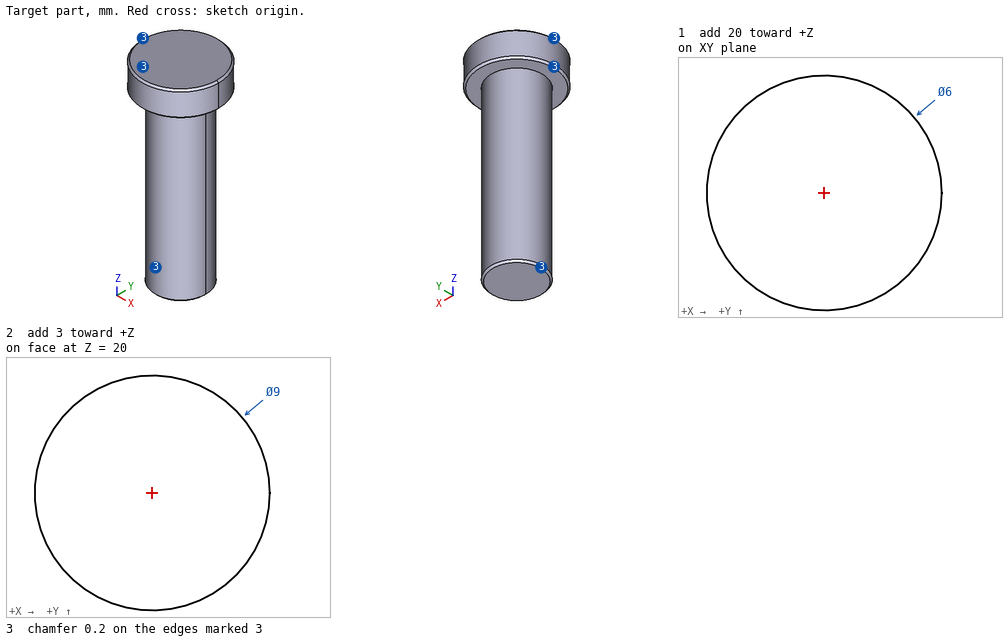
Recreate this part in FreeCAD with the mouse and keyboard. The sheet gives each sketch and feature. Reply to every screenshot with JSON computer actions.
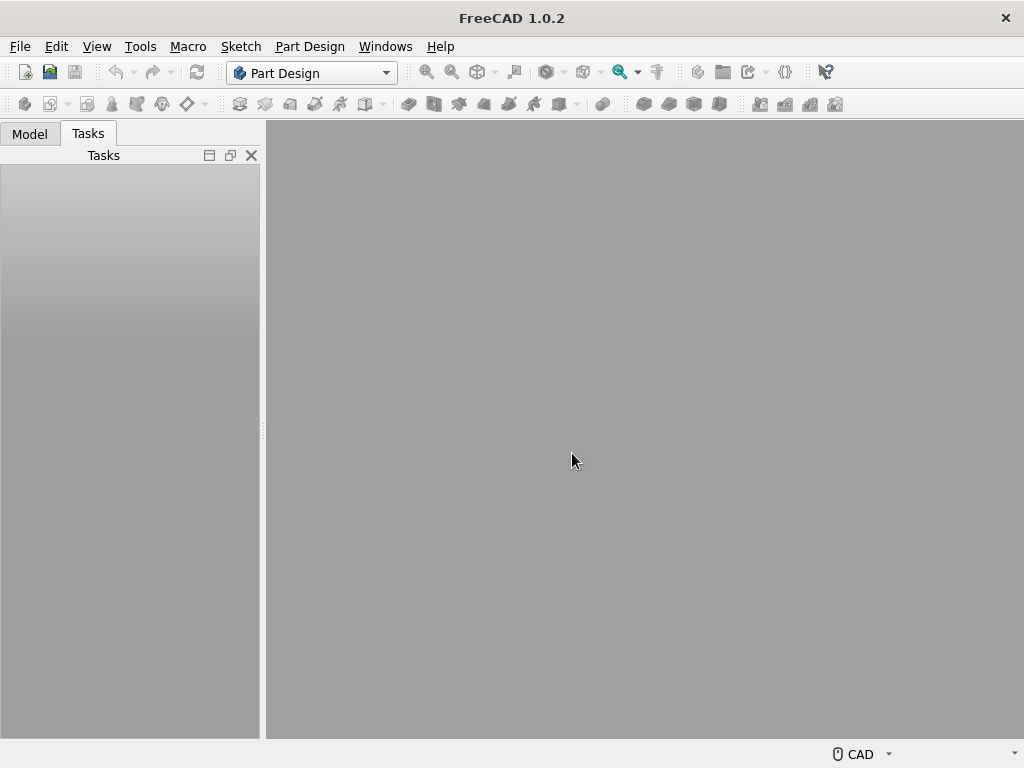
{"action": "left_click", "coordinate": [25, 72]}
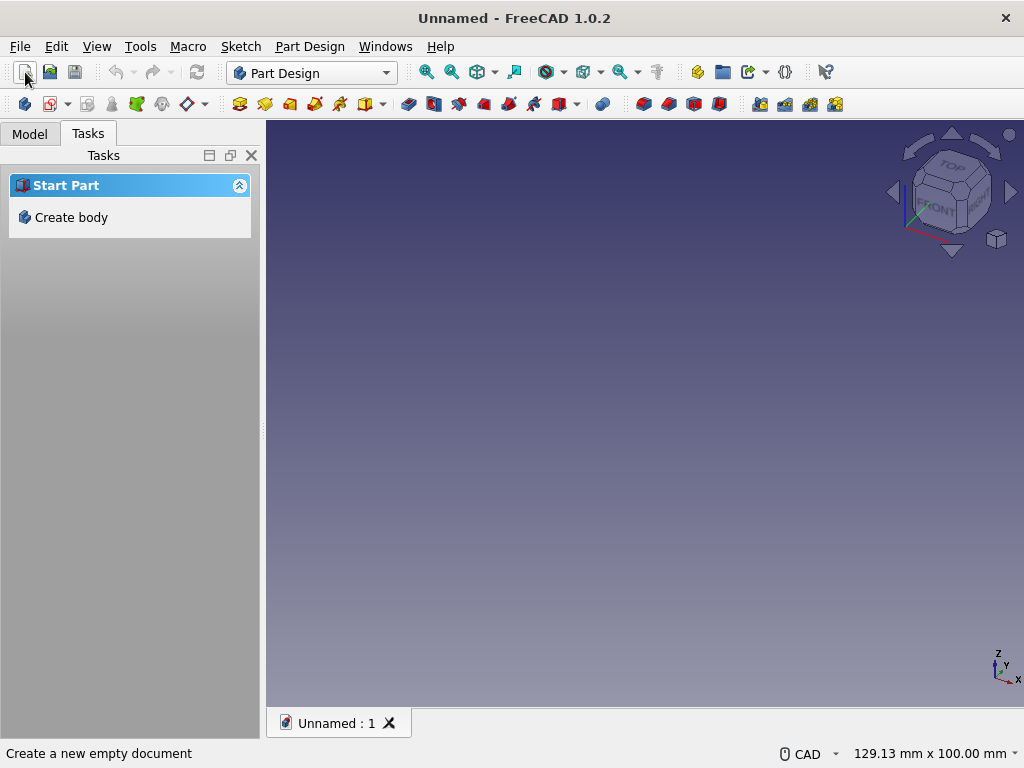
{"action": "left_click", "coordinate": [50, 104]}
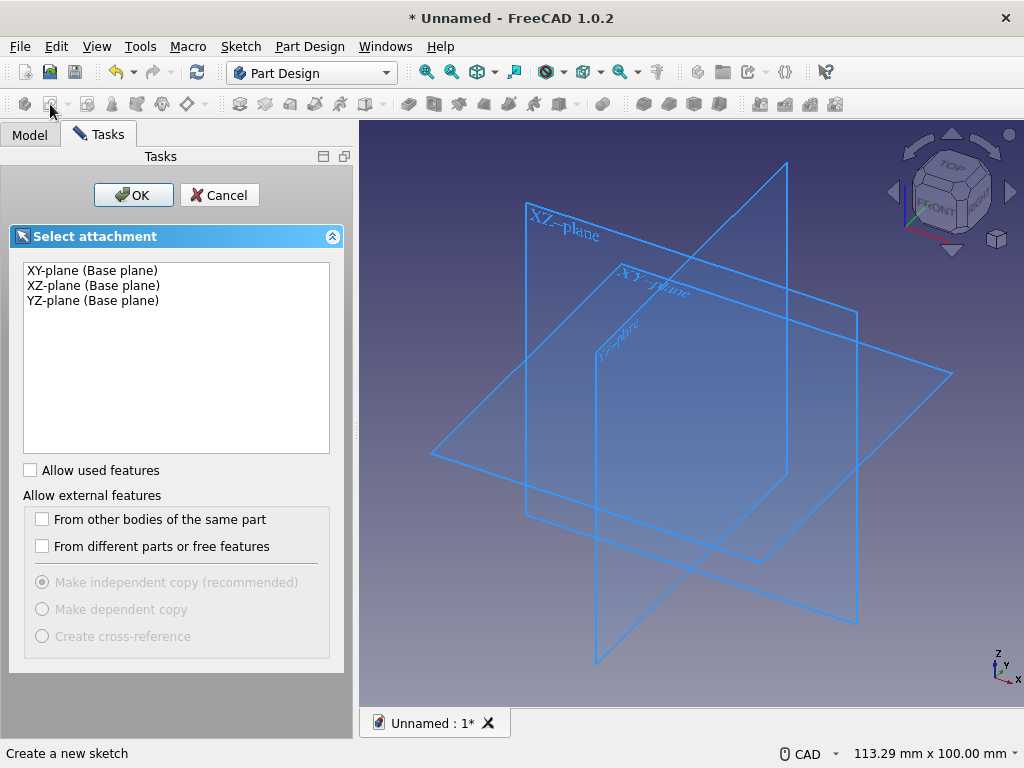
{"action": "left_click", "coordinate": [84, 270]}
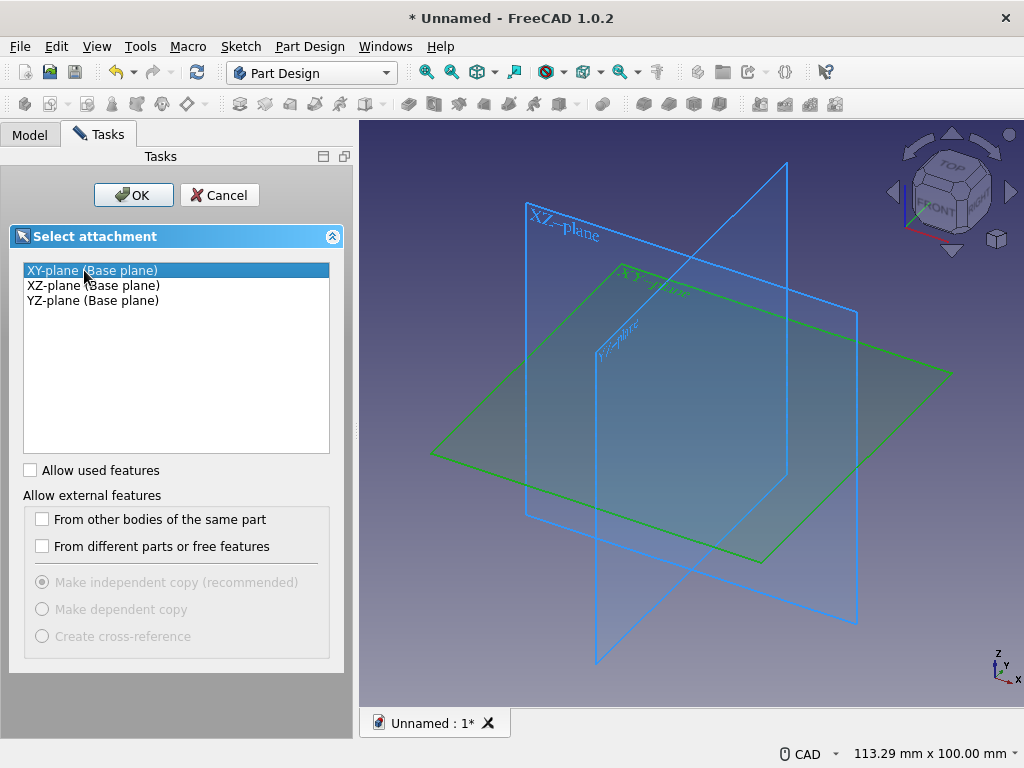
{"action": "left_click", "coordinate": [134, 195]}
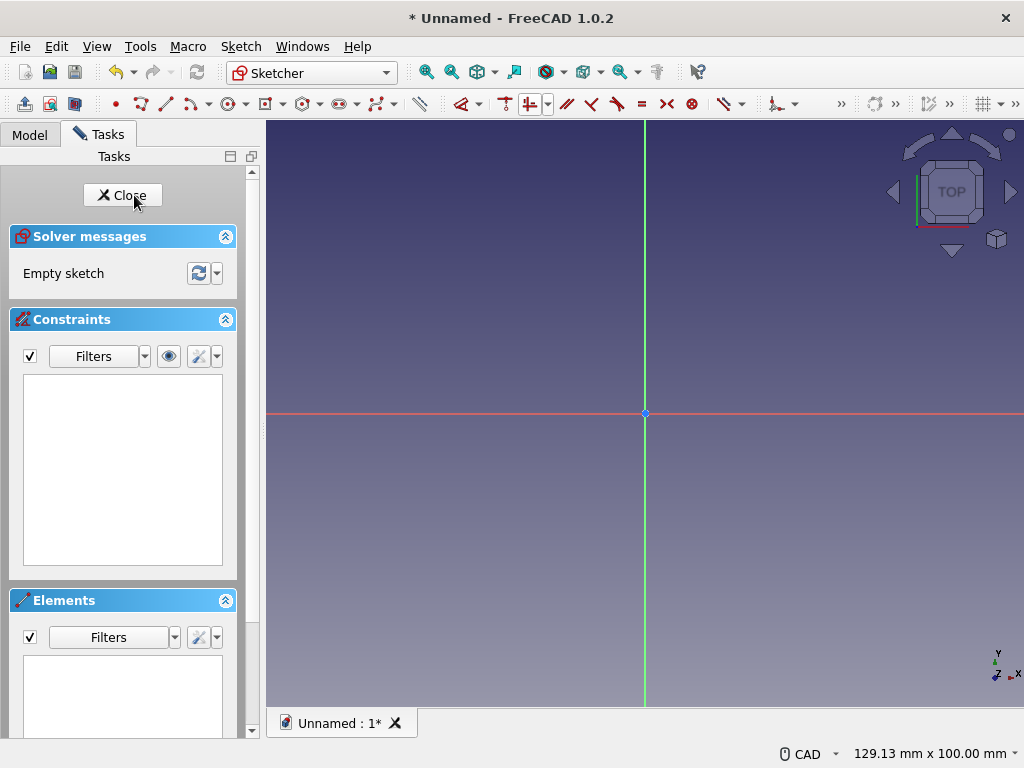
{"action": "scroll", "coordinate": [652, 414], "scroll_direction": "up", "scroll_amount": 12}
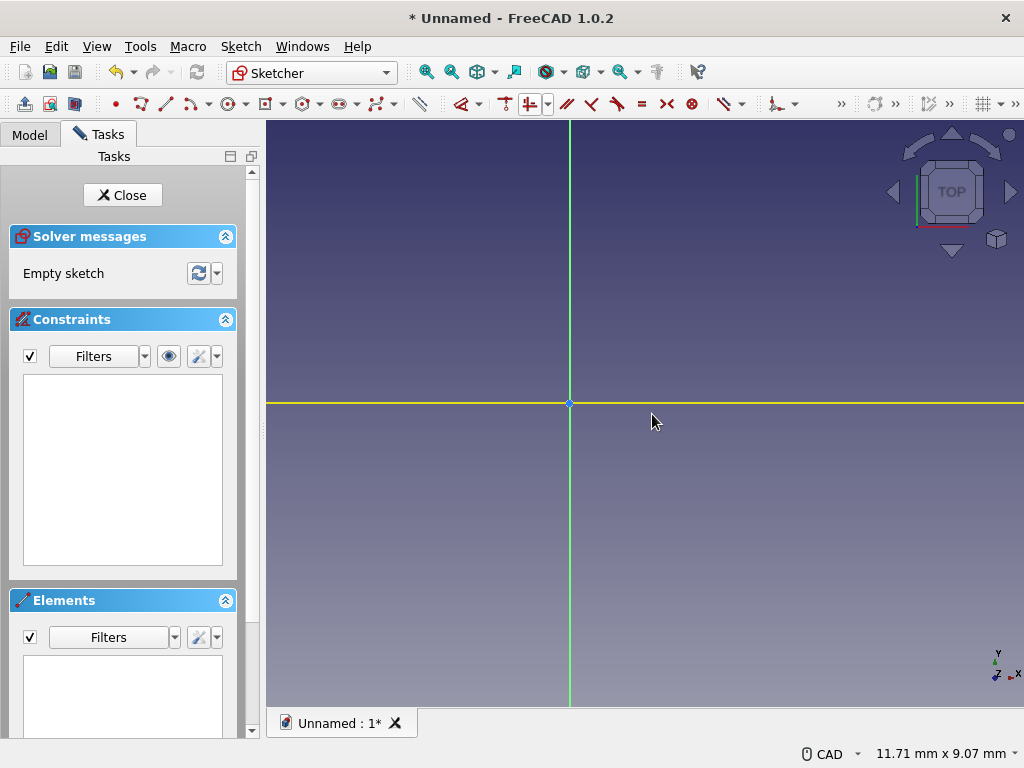
{"action": "key", "text": "g c"}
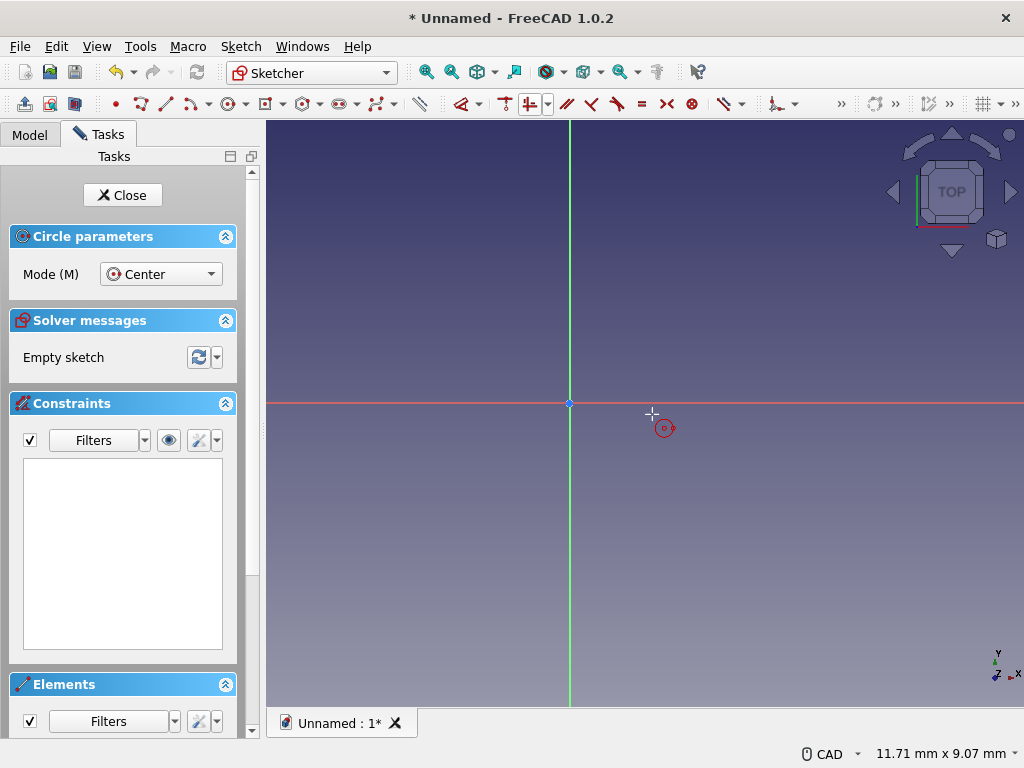
{"action": "left_click", "coordinate": [570, 403]}
{"action": "mouse_move", "coordinate": [707, 266]}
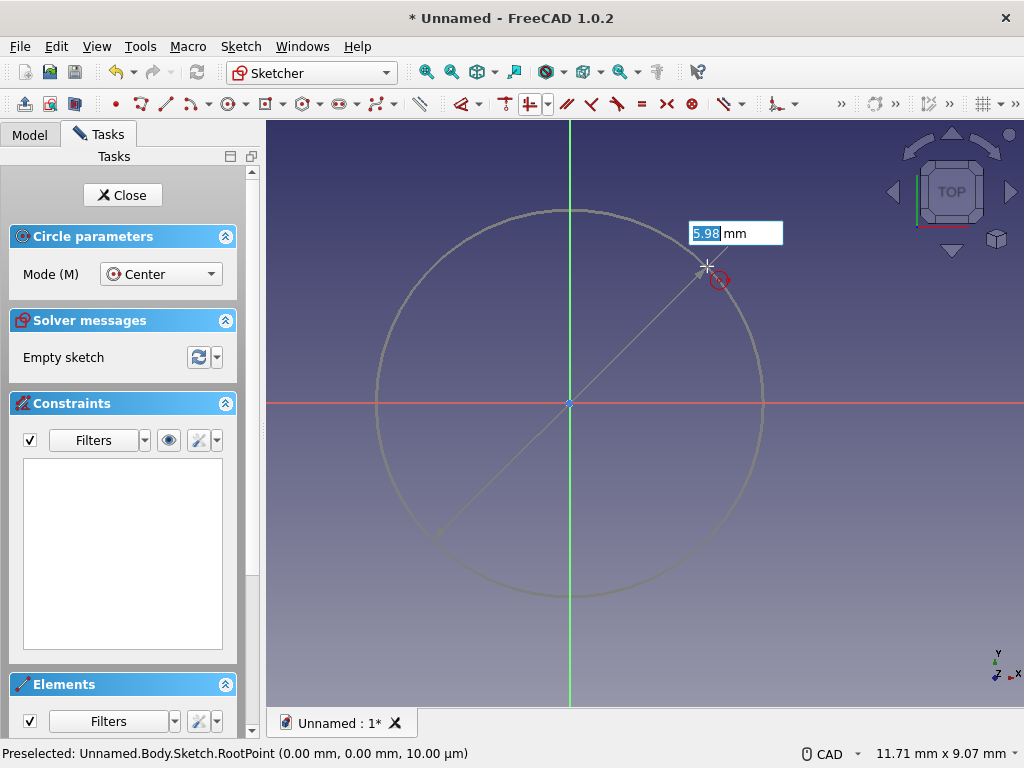
{"action": "type", "text": "6"}
{"action": "key", "text": "Return"}
{"action": "key", "text": "Escape"}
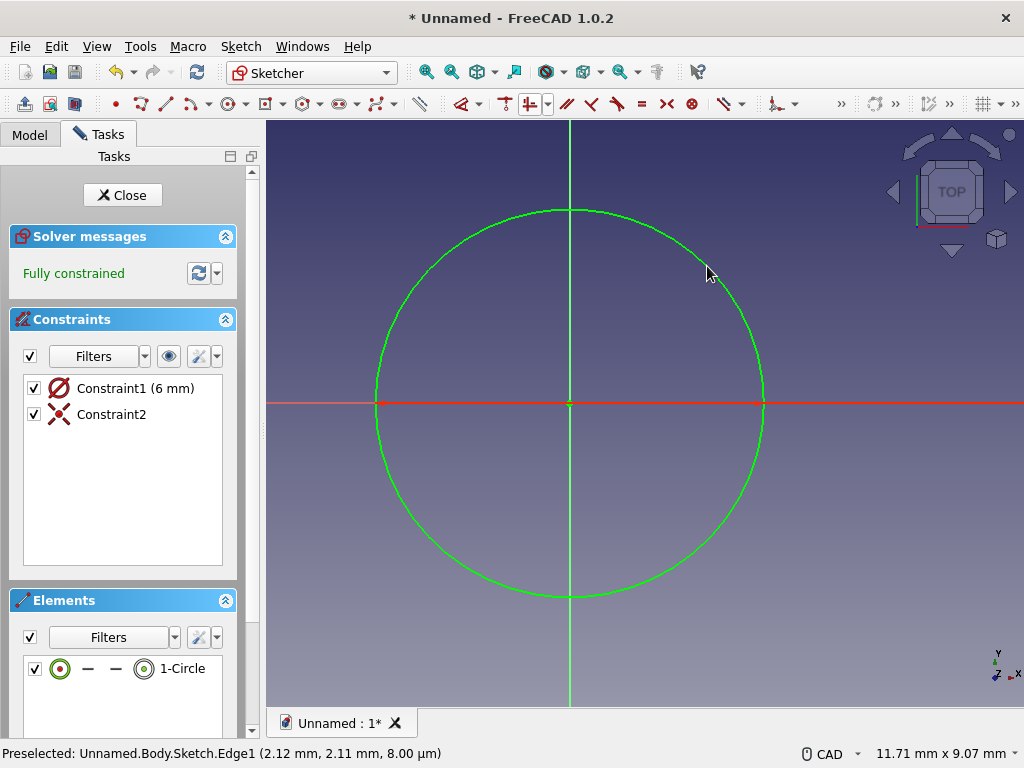
{"action": "left_click", "coordinate": [123, 195]}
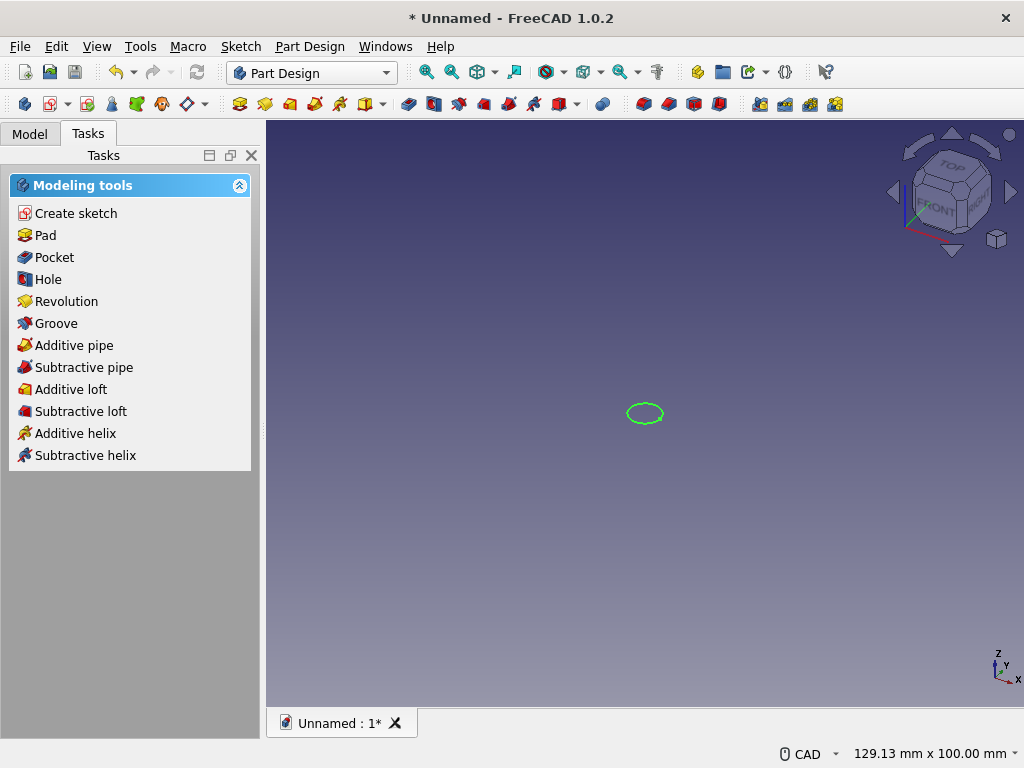
{"action": "left_click", "coordinate": [240, 104]}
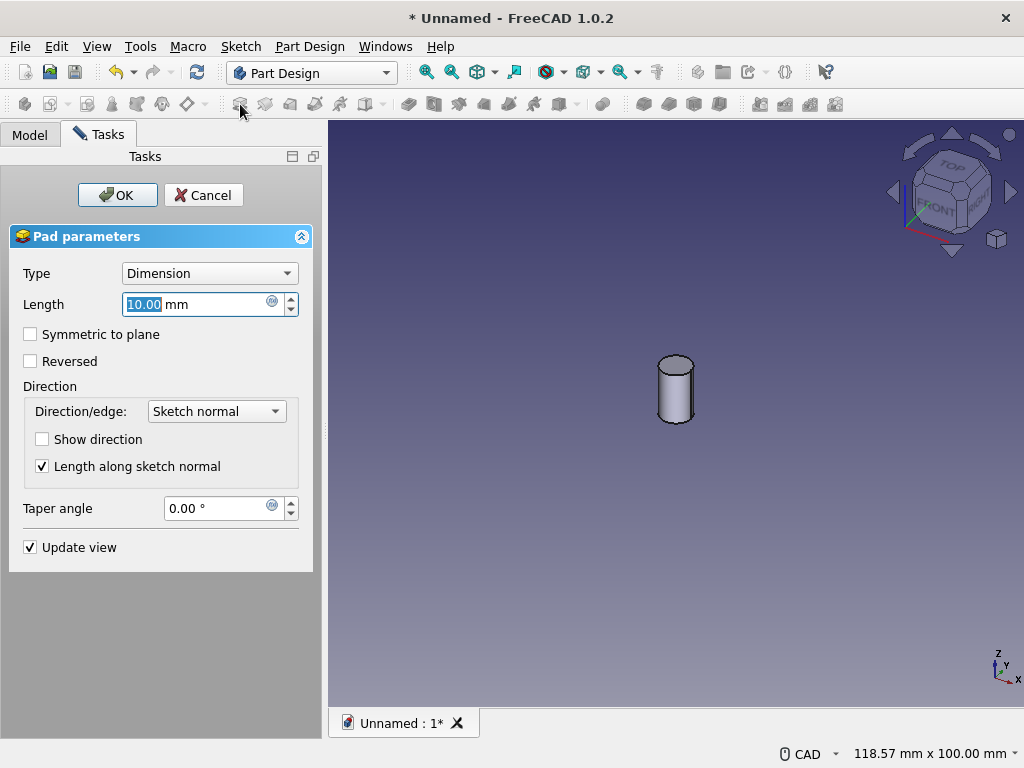
{"action": "type", "text": "20"}
{"action": "key", "text": "Tab"}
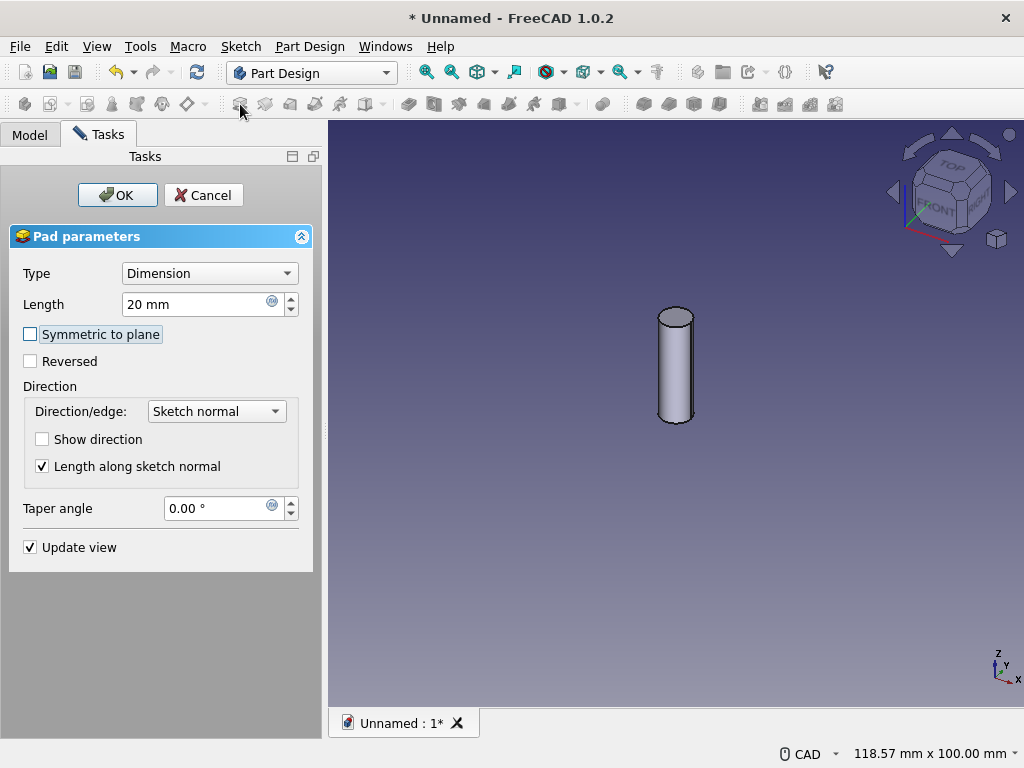
{"action": "left_click", "coordinate": [118, 195]}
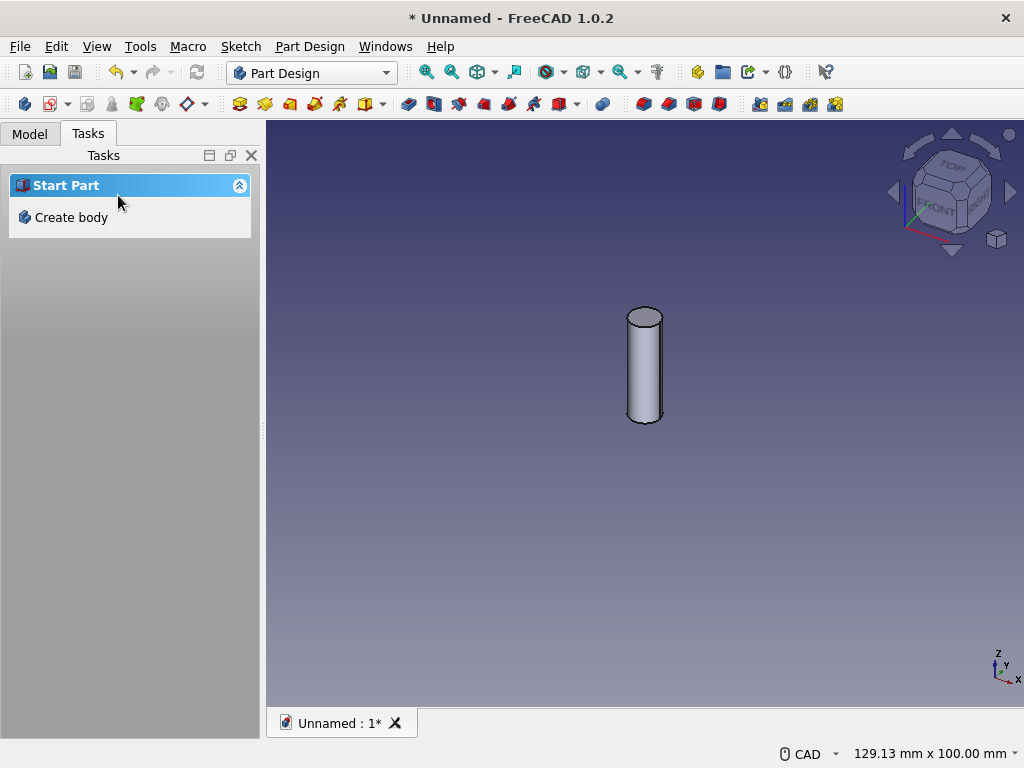
{"action": "key", "text": "v f"}